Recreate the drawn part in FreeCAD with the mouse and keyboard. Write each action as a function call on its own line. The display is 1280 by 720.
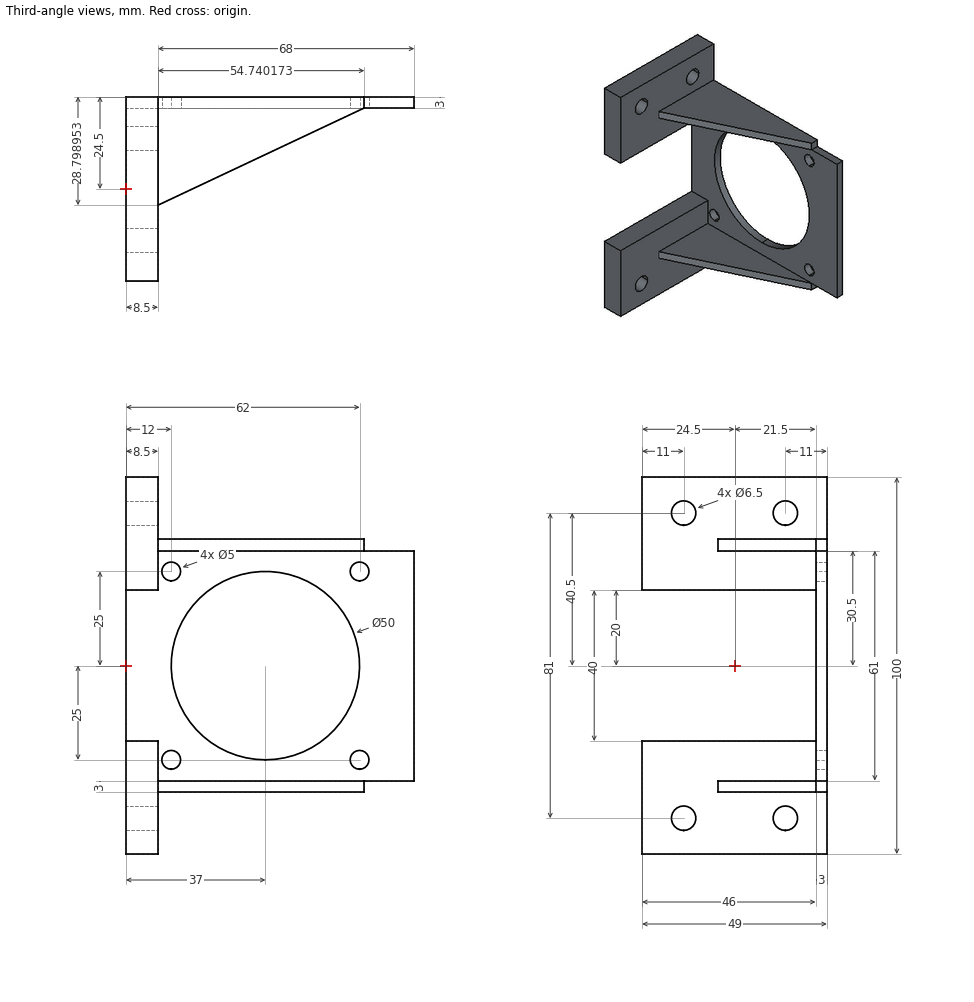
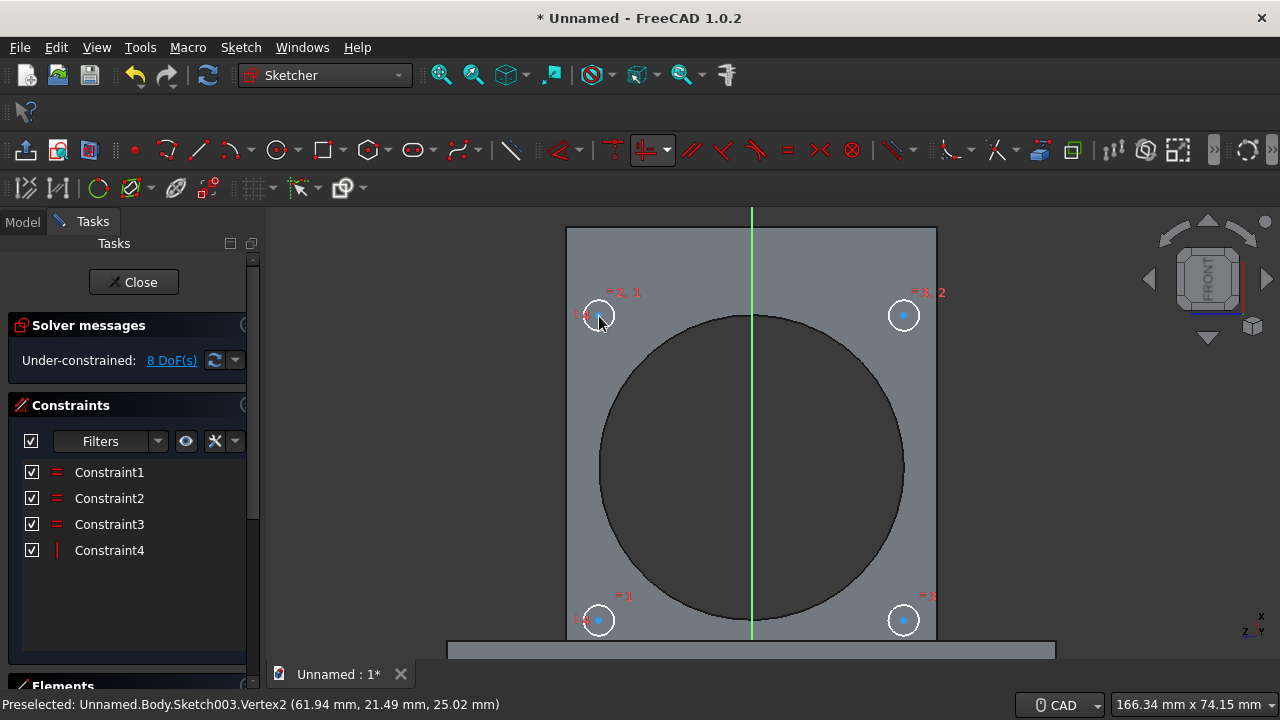
click(599, 316)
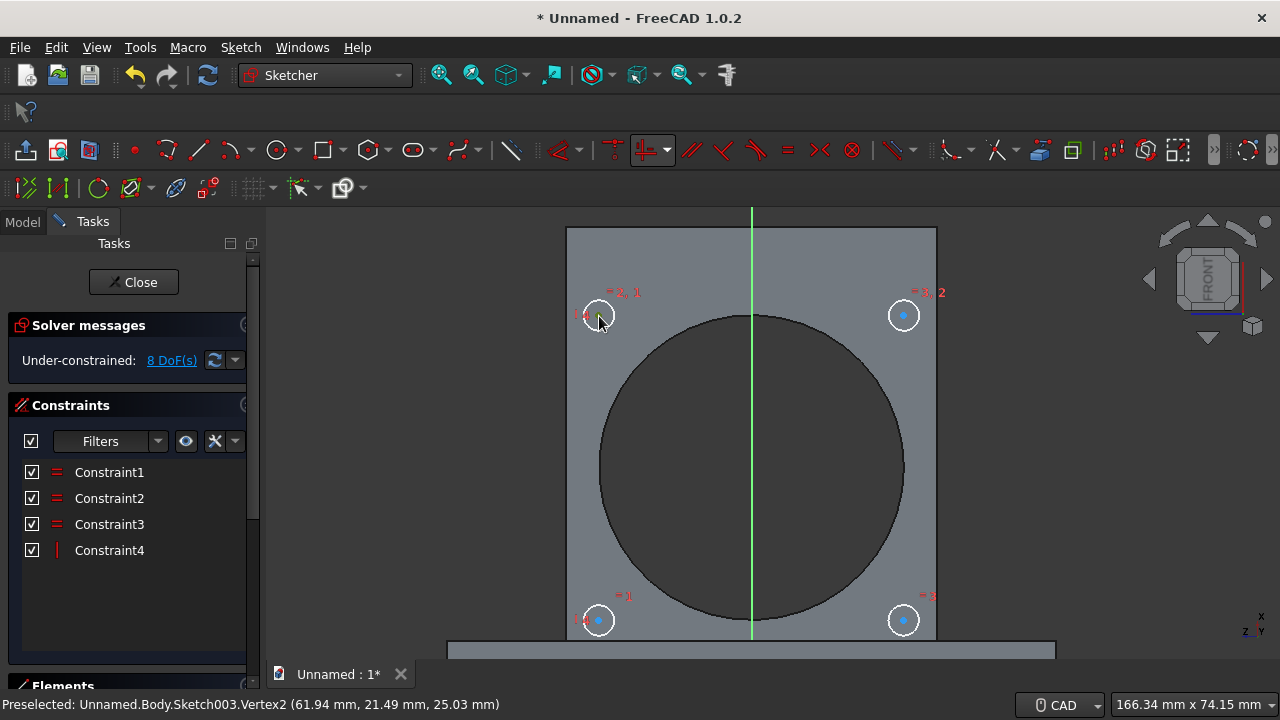
click(904, 316)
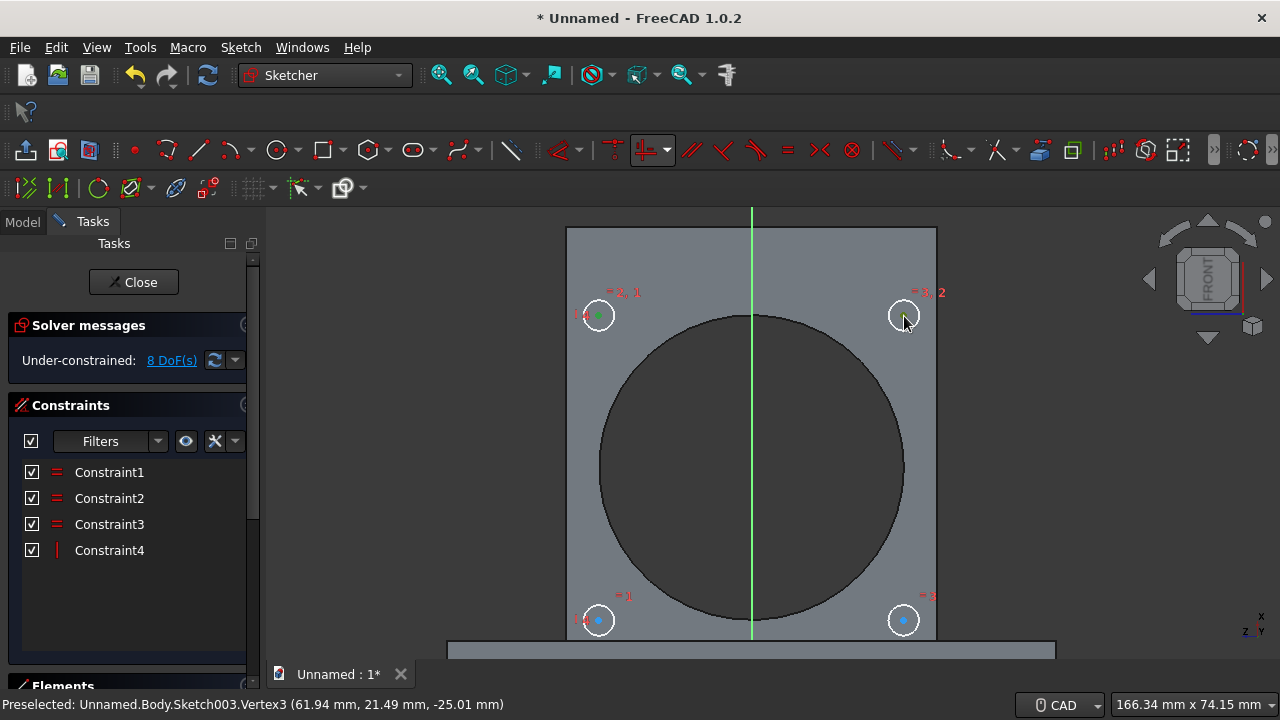
click(670, 150)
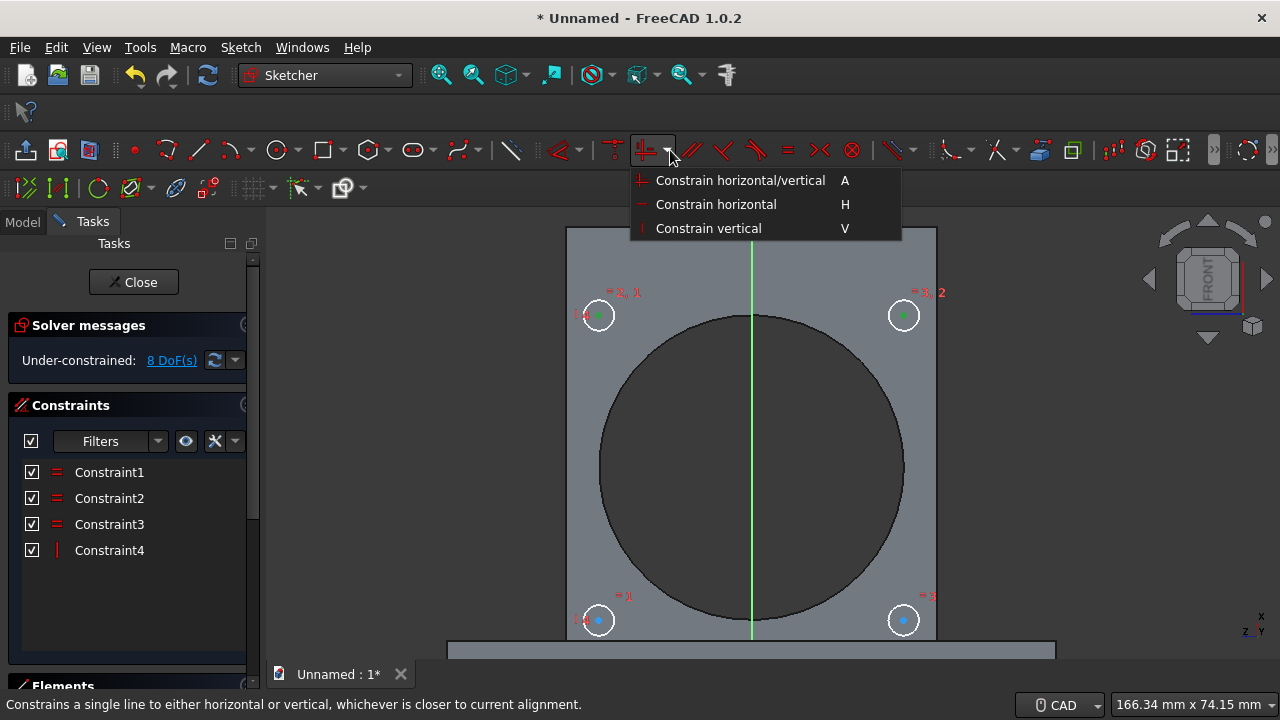
click(766, 204)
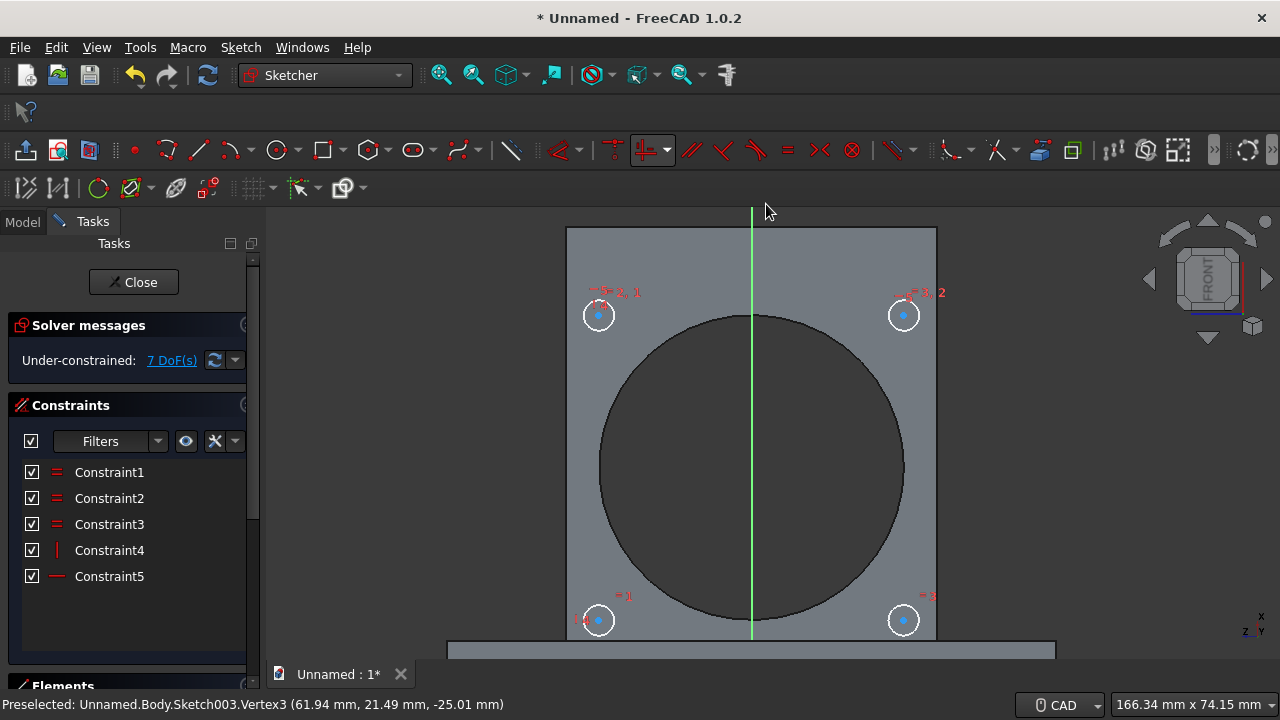
click(904, 316)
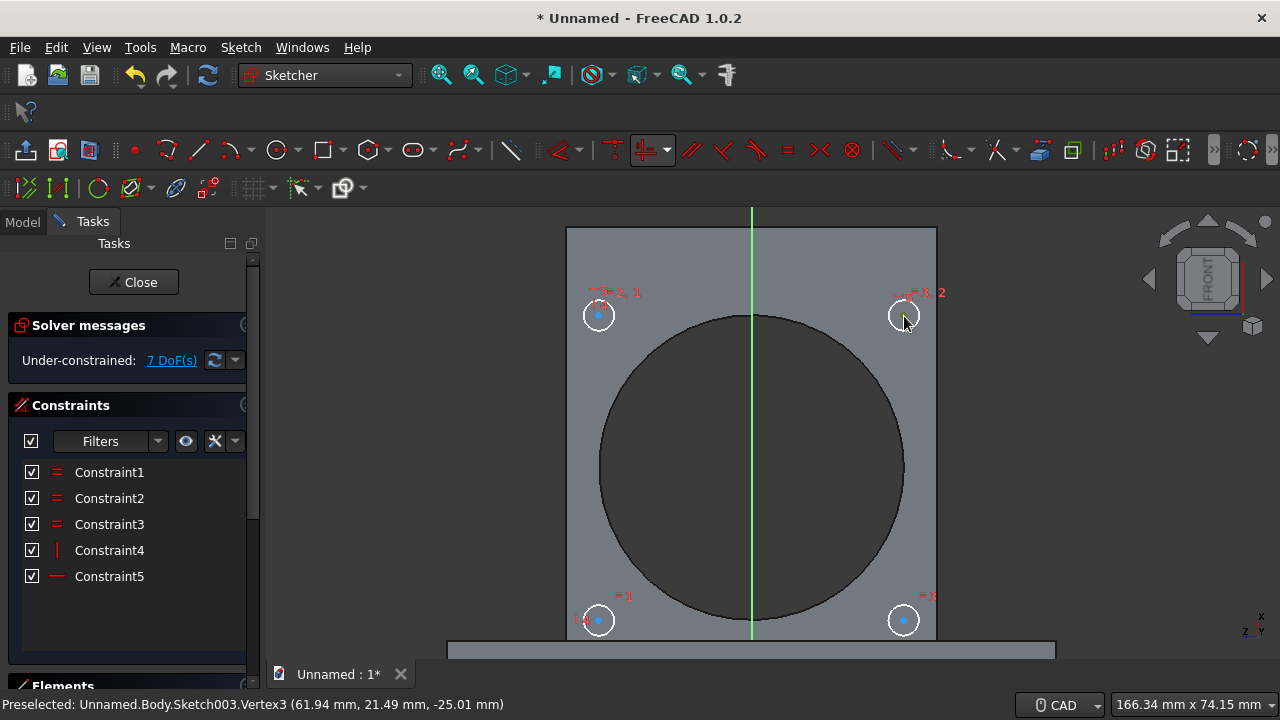
click(904, 620)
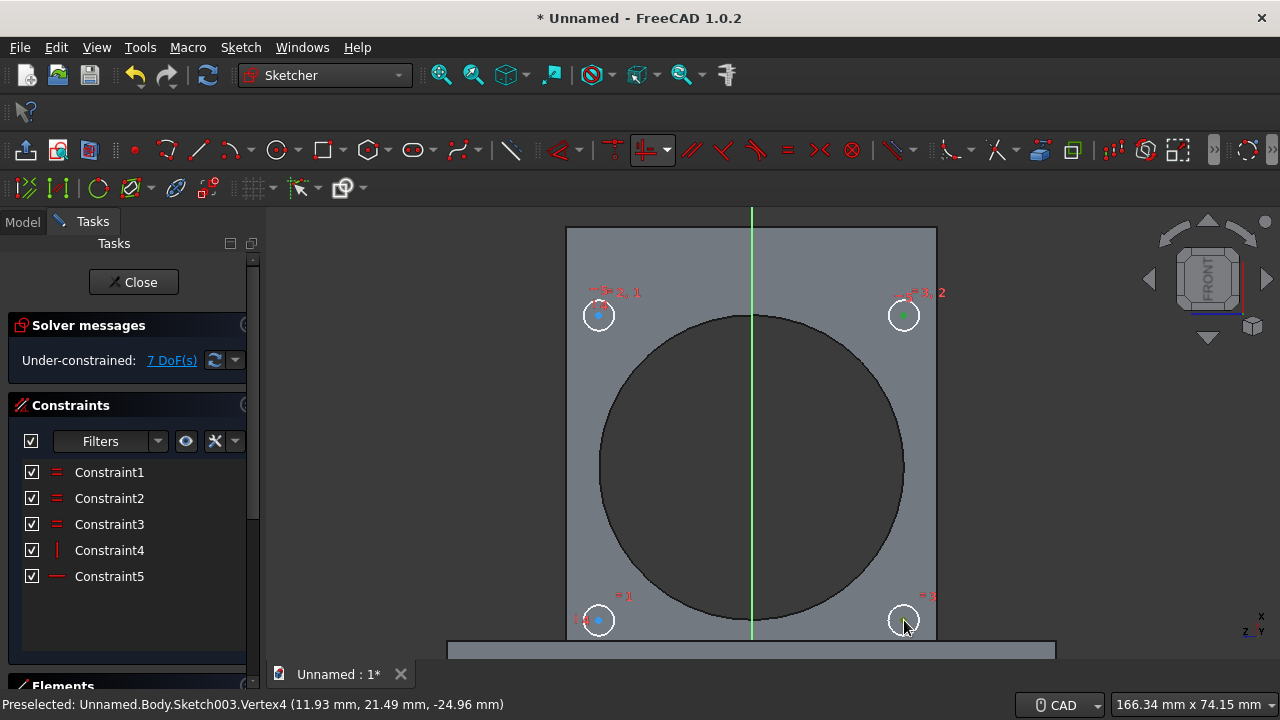
click(670, 150)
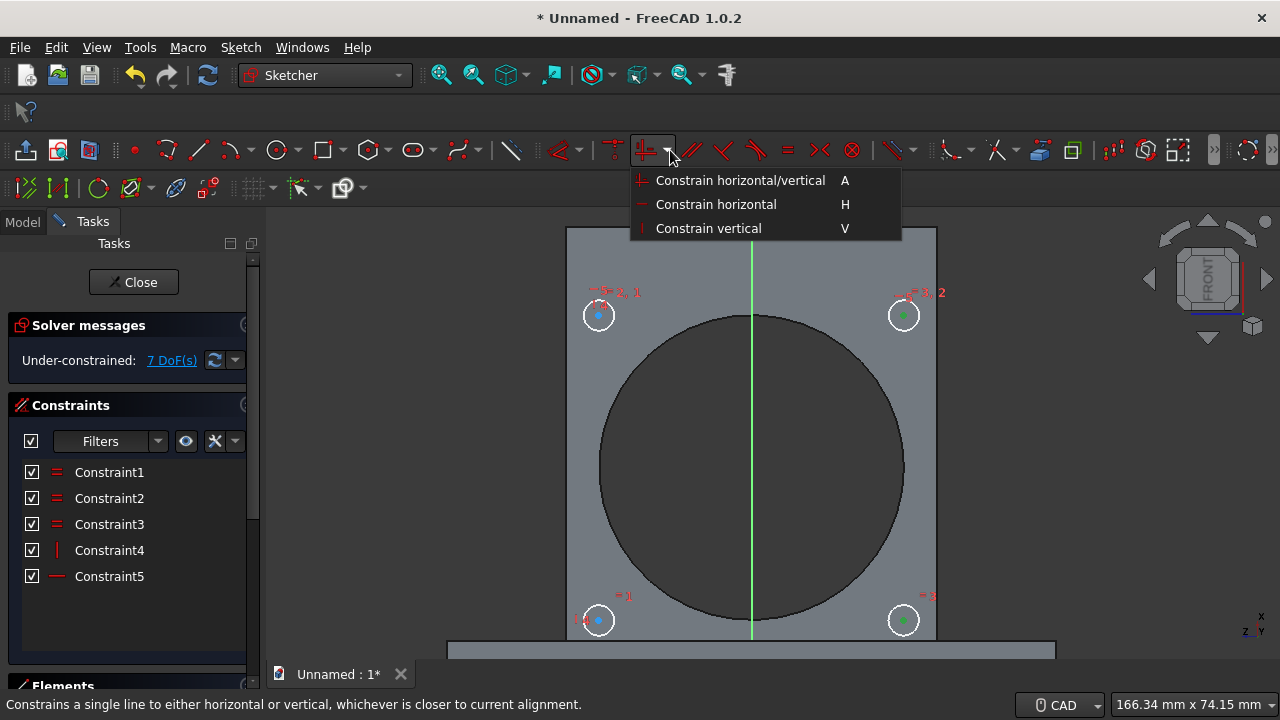
click(766, 228)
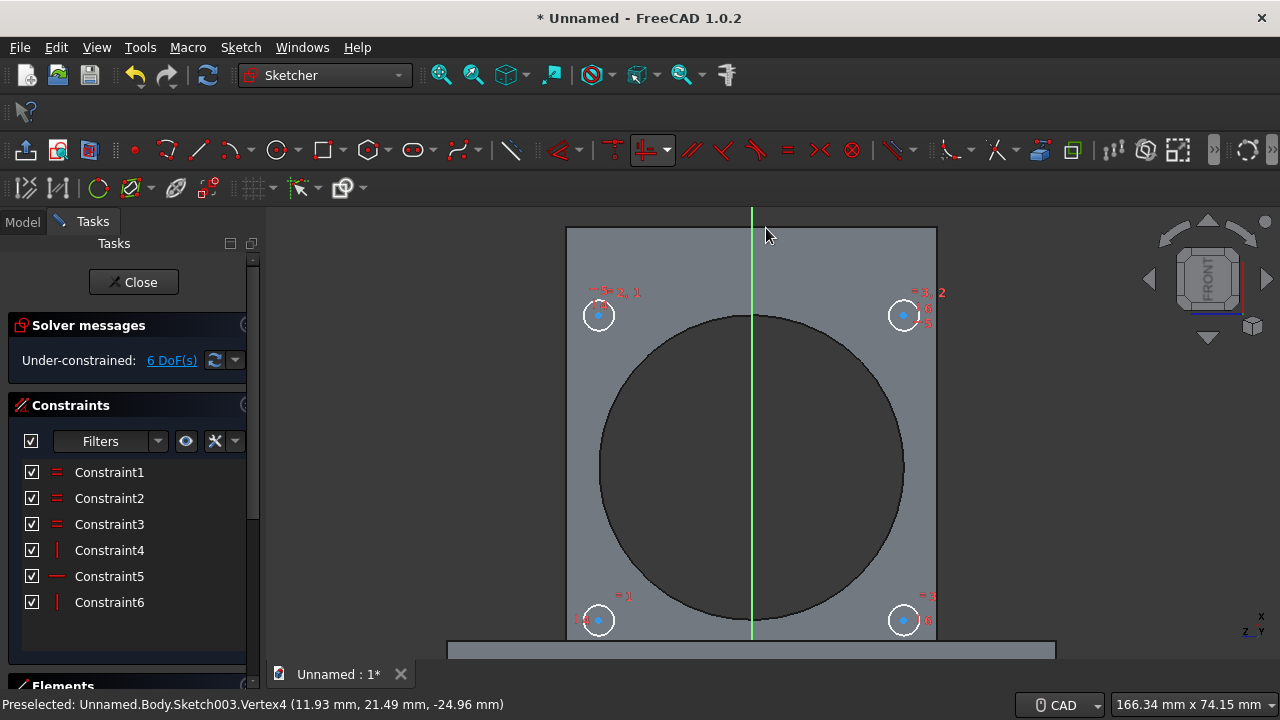
click(599, 620)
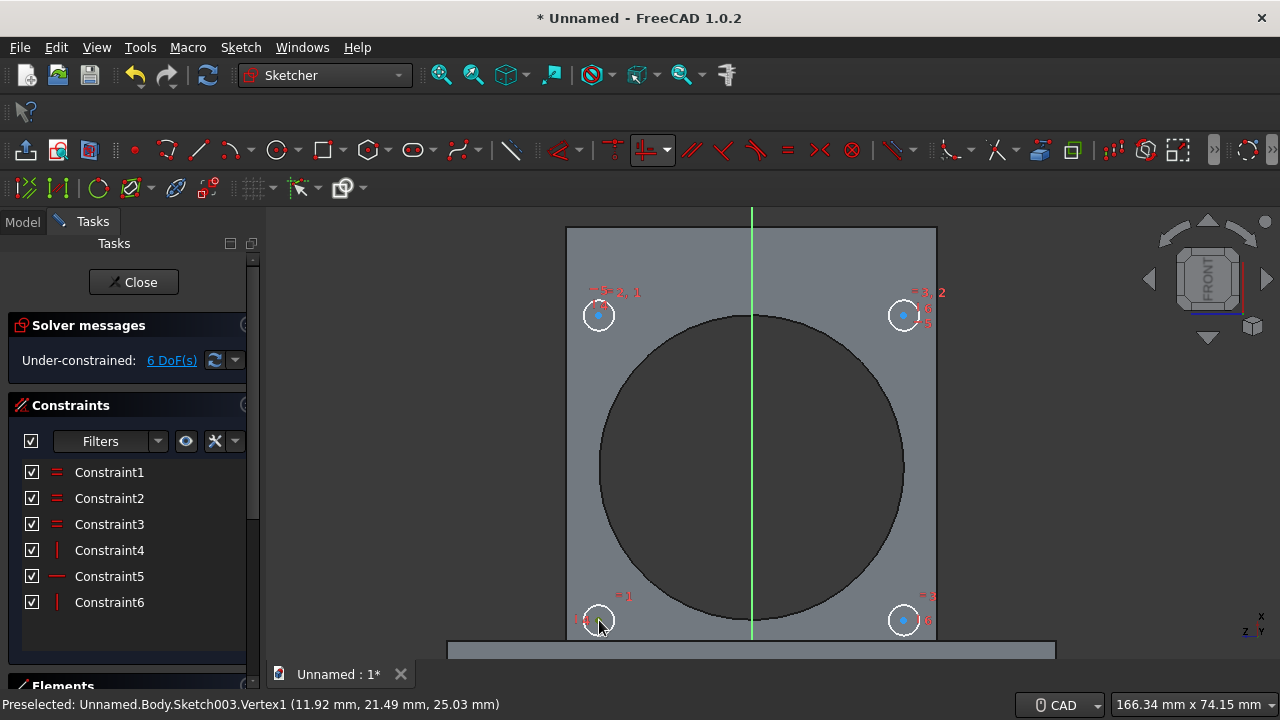
click(904, 620)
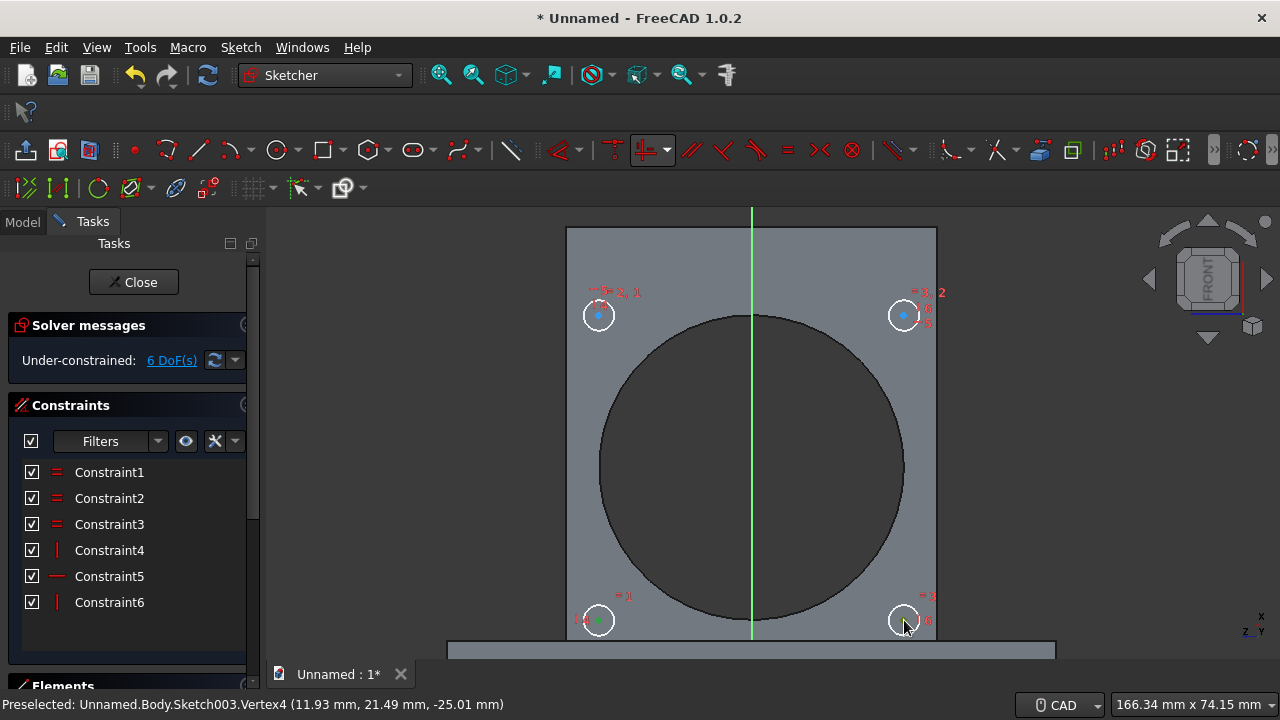
key(h)